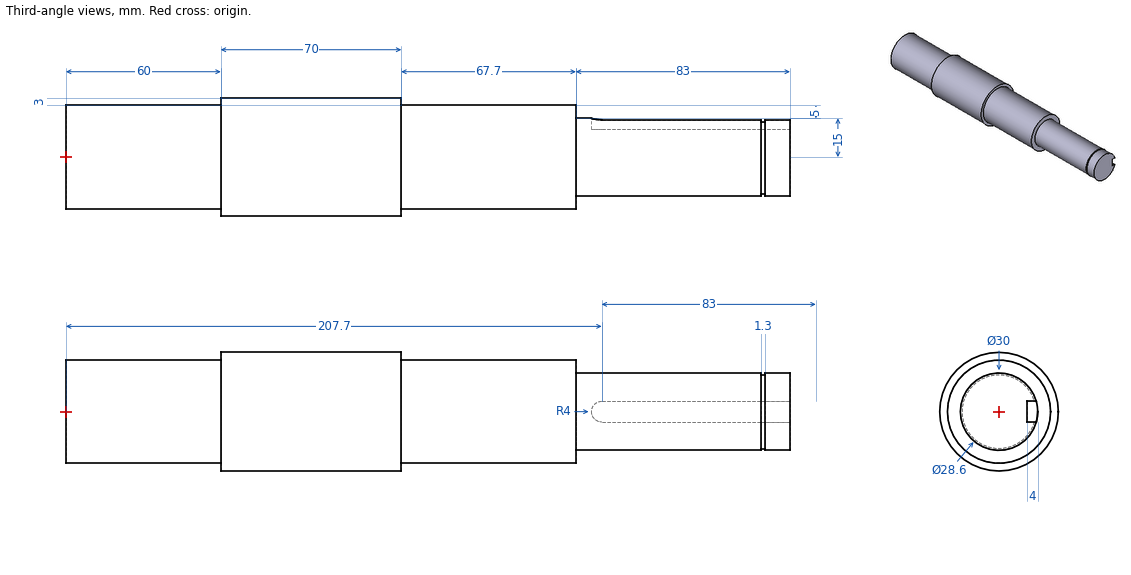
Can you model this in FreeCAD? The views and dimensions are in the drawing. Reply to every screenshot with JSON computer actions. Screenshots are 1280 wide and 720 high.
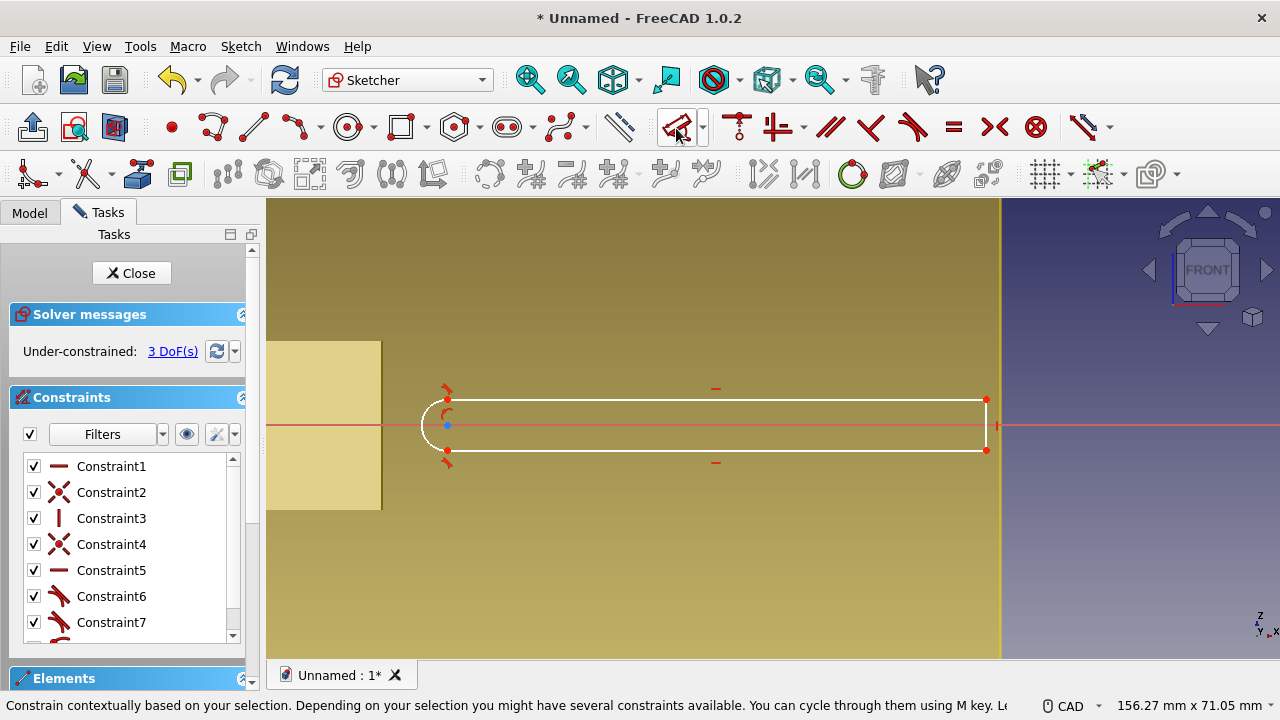
{"action": "scroll", "coordinate": [427, 410], "scroll_direction": "up", "scroll_amount": 3}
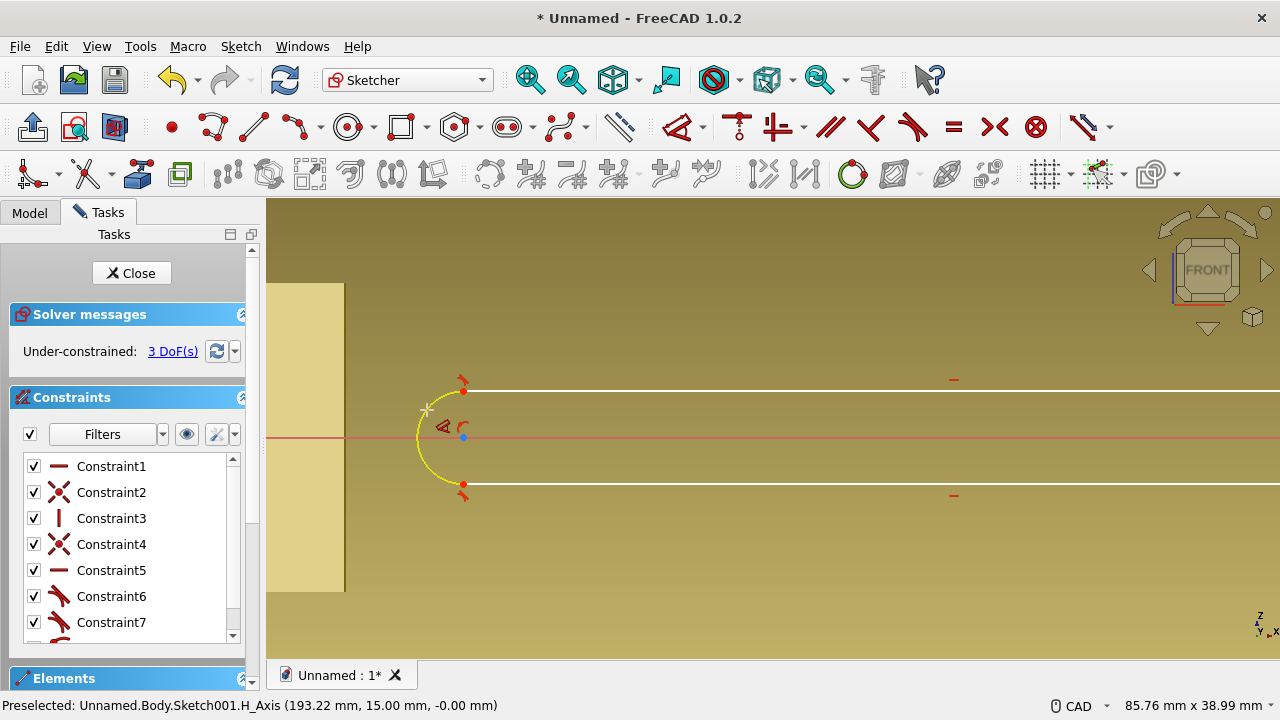
{"action": "left_click", "coordinate": [426, 411]}
{"action": "left_click", "coordinate": [400, 392]}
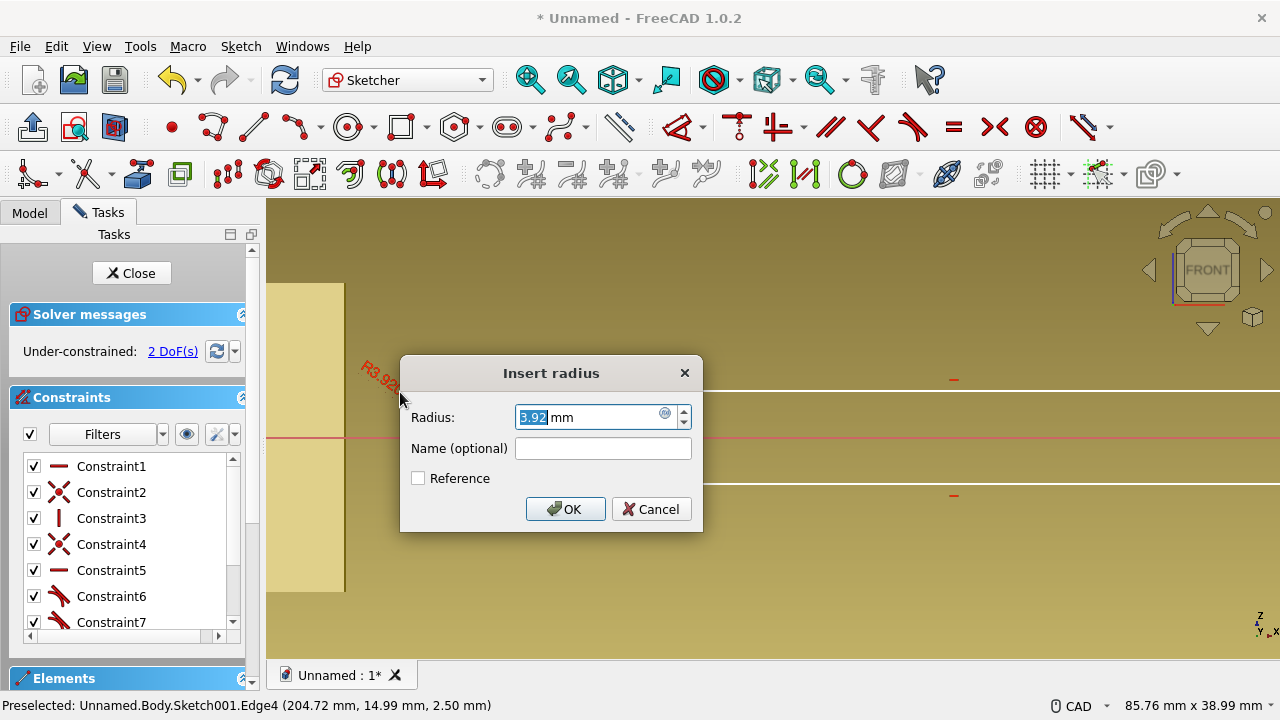
{"action": "type", "text": "4"}
{"action": "key", "text": "Return"}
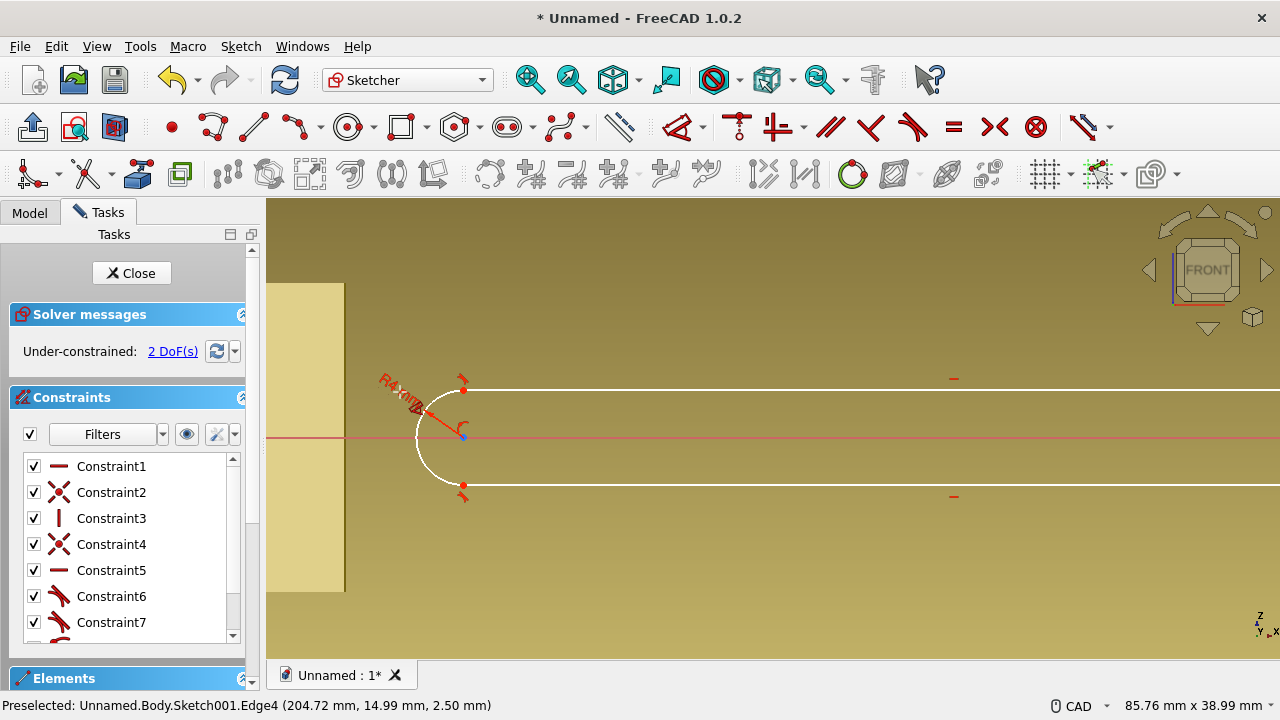
{"action": "left_click", "coordinate": [758, 390]}
{"action": "left_click", "coordinate": [789, 356]}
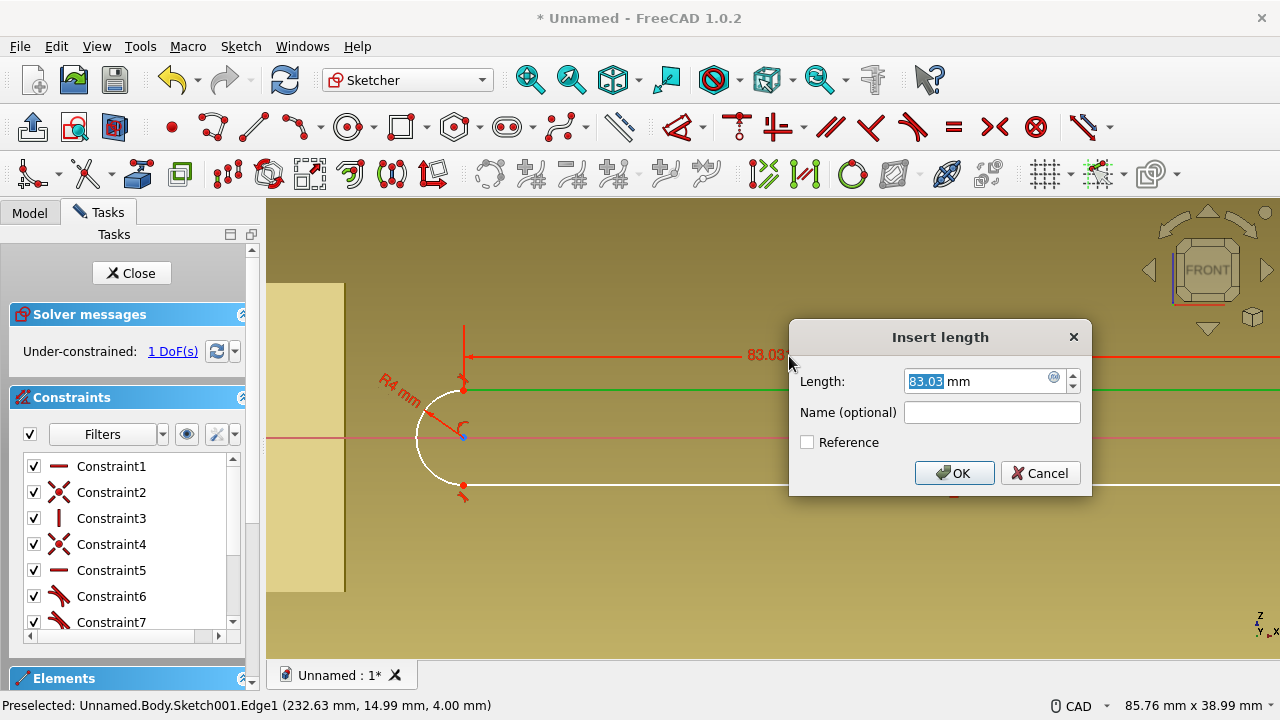
{"action": "type", "text": "83"}
{"action": "key", "text": "Return"}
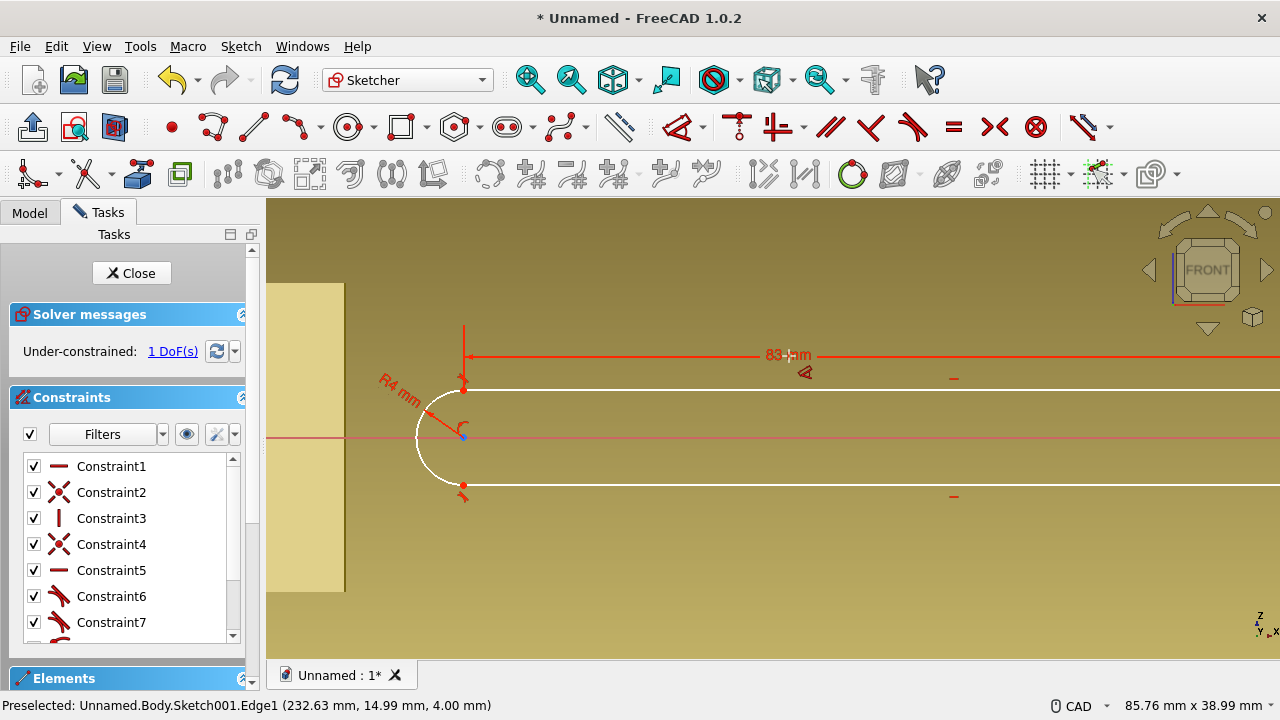
{"action": "left_click", "coordinate": [464, 390]}
{"action": "left_click", "coordinate": [379, 356]}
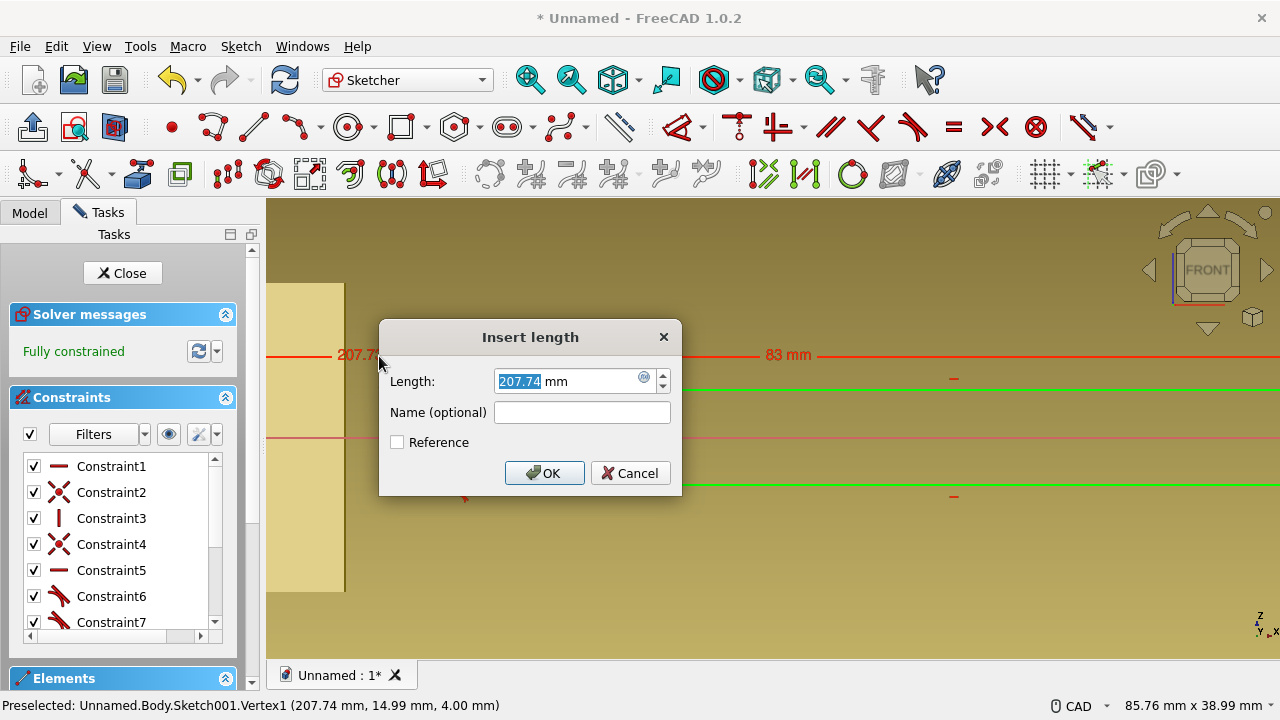
{"action": "type", "text": "207.7"}
{"action": "key", "text": "Return"}
{"action": "key", "text": "Escape"}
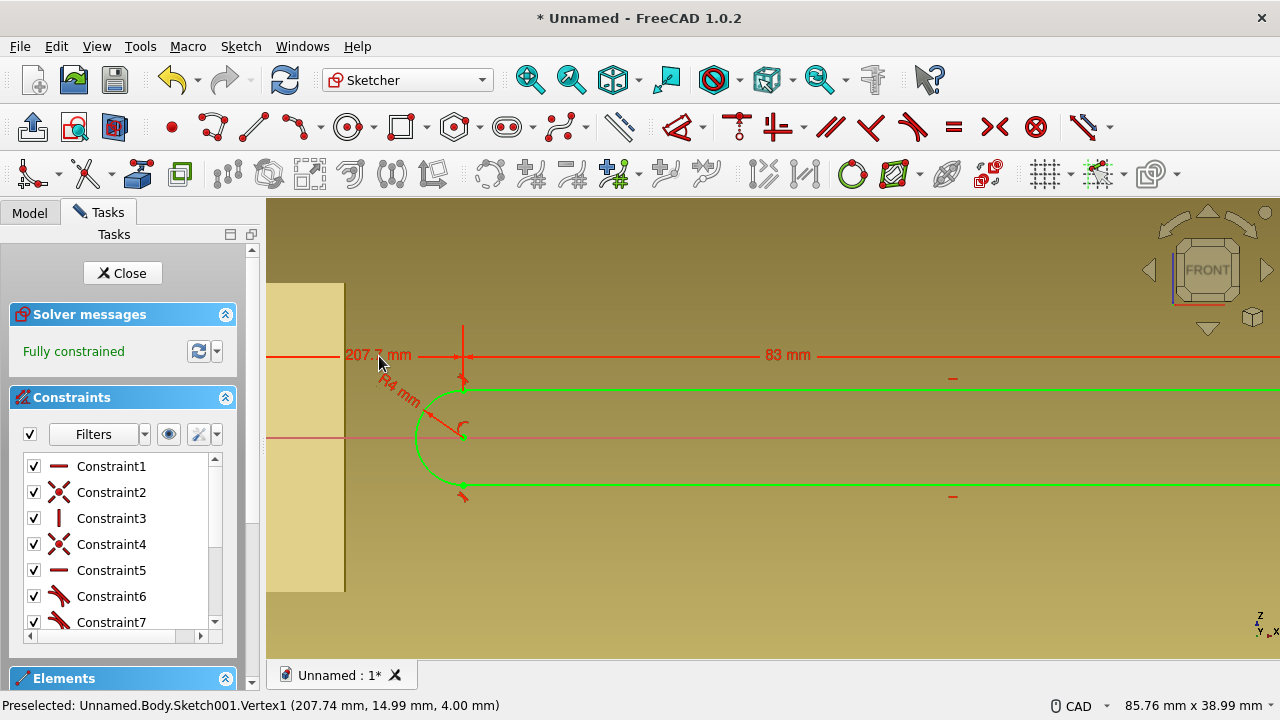
{"action": "left_click", "coordinate": [123, 273]}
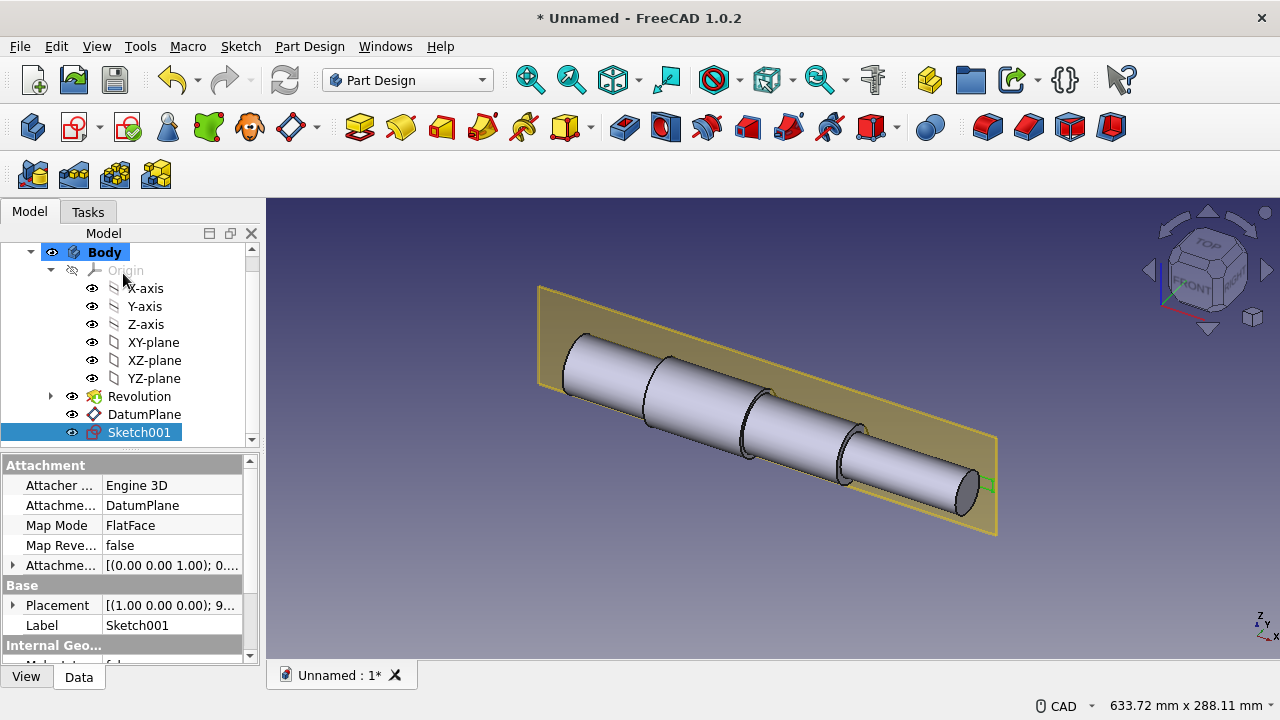
{"action": "left_click", "coordinate": [625, 128]}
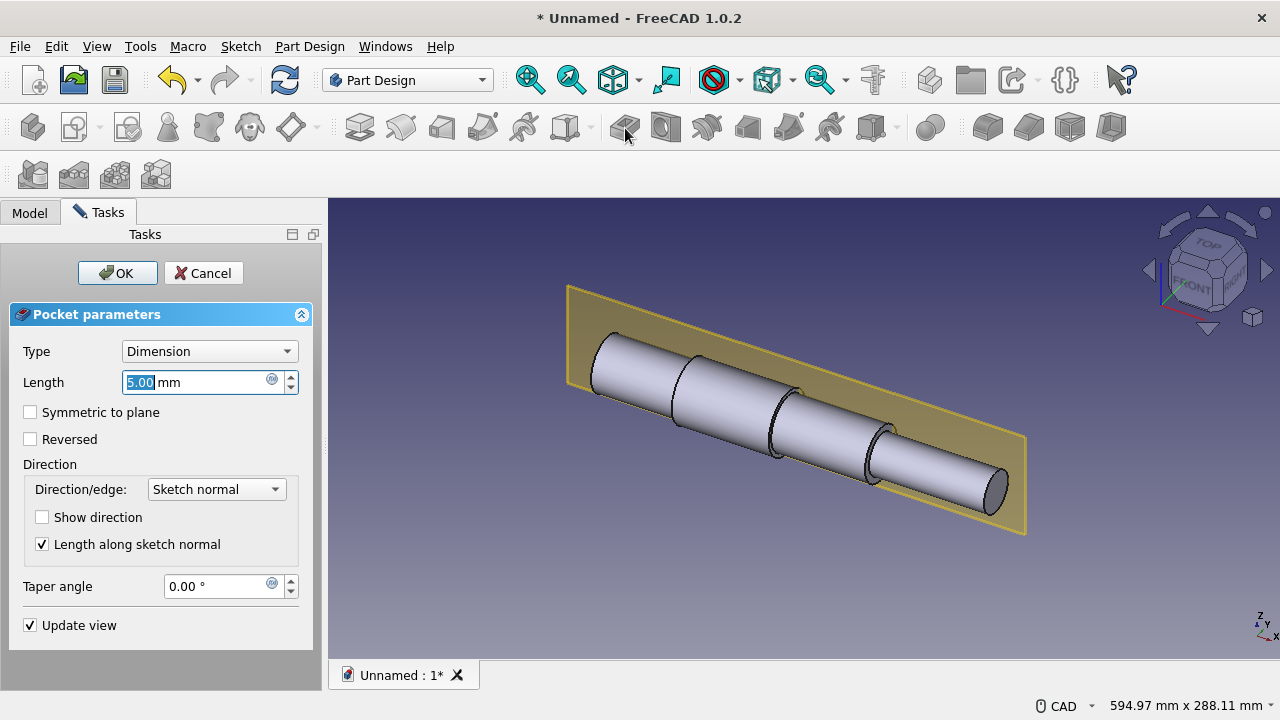
{"action": "type", "text": "4"}
{"action": "key", "text": "Tab"}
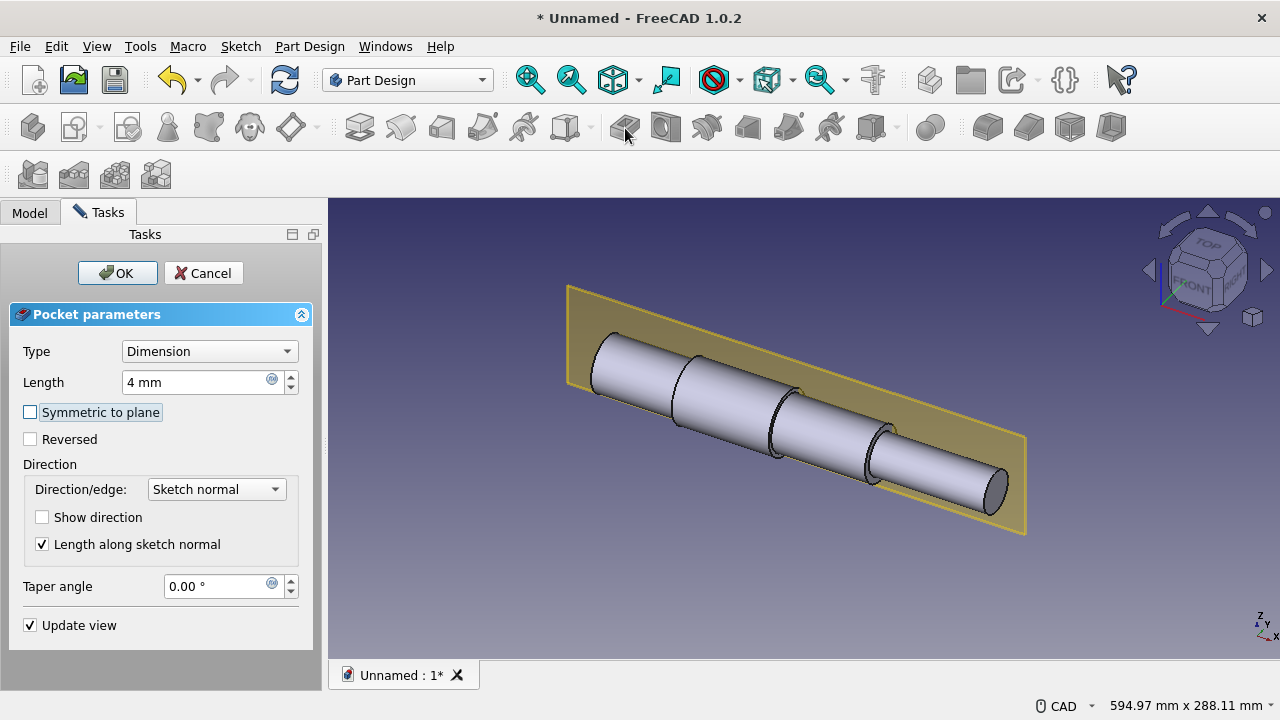
{"action": "left_click", "coordinate": [31, 439]}